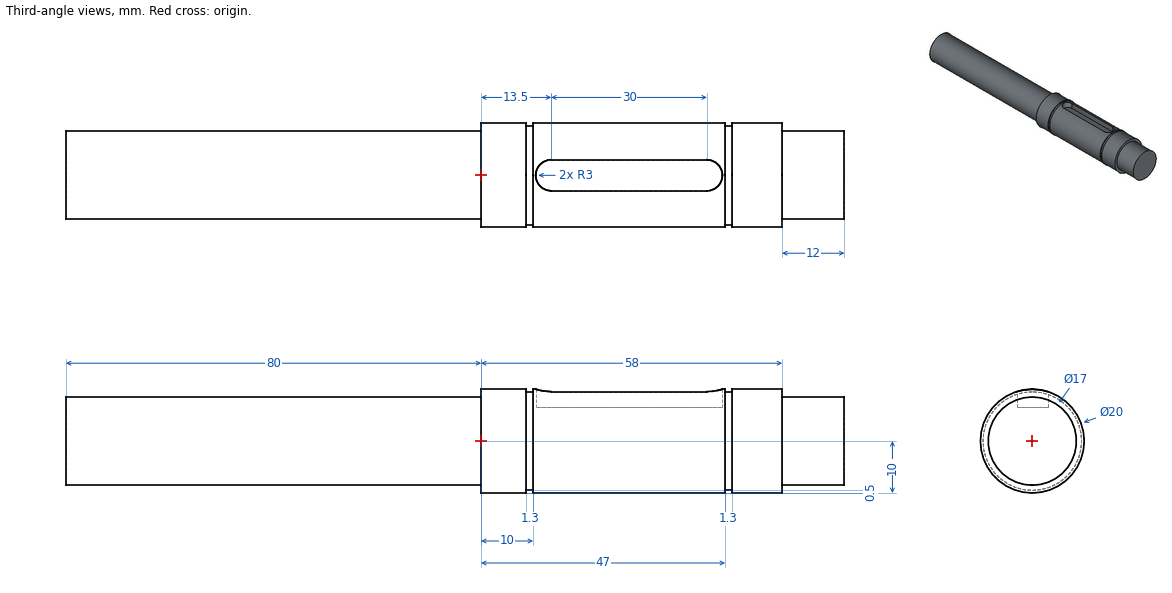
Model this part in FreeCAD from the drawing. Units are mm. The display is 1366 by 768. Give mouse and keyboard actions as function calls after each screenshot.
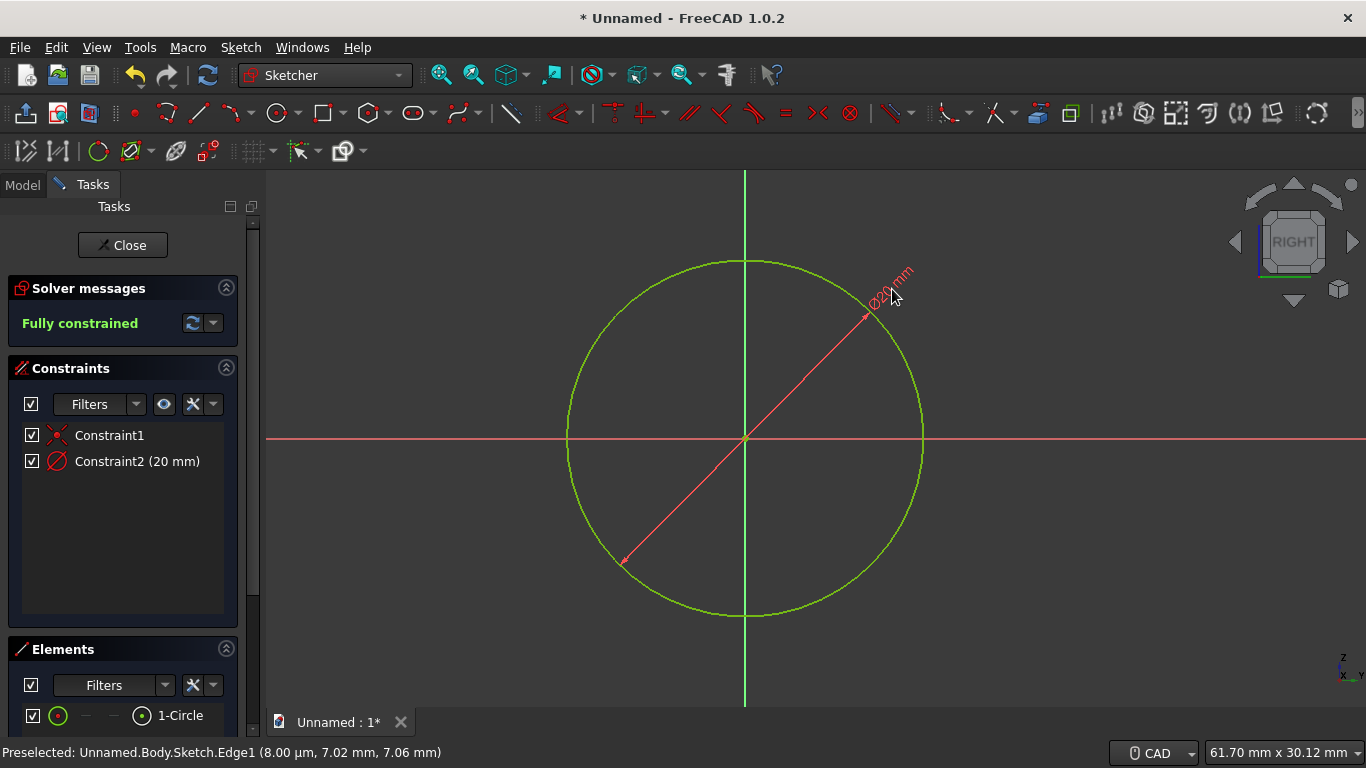
click(123, 245)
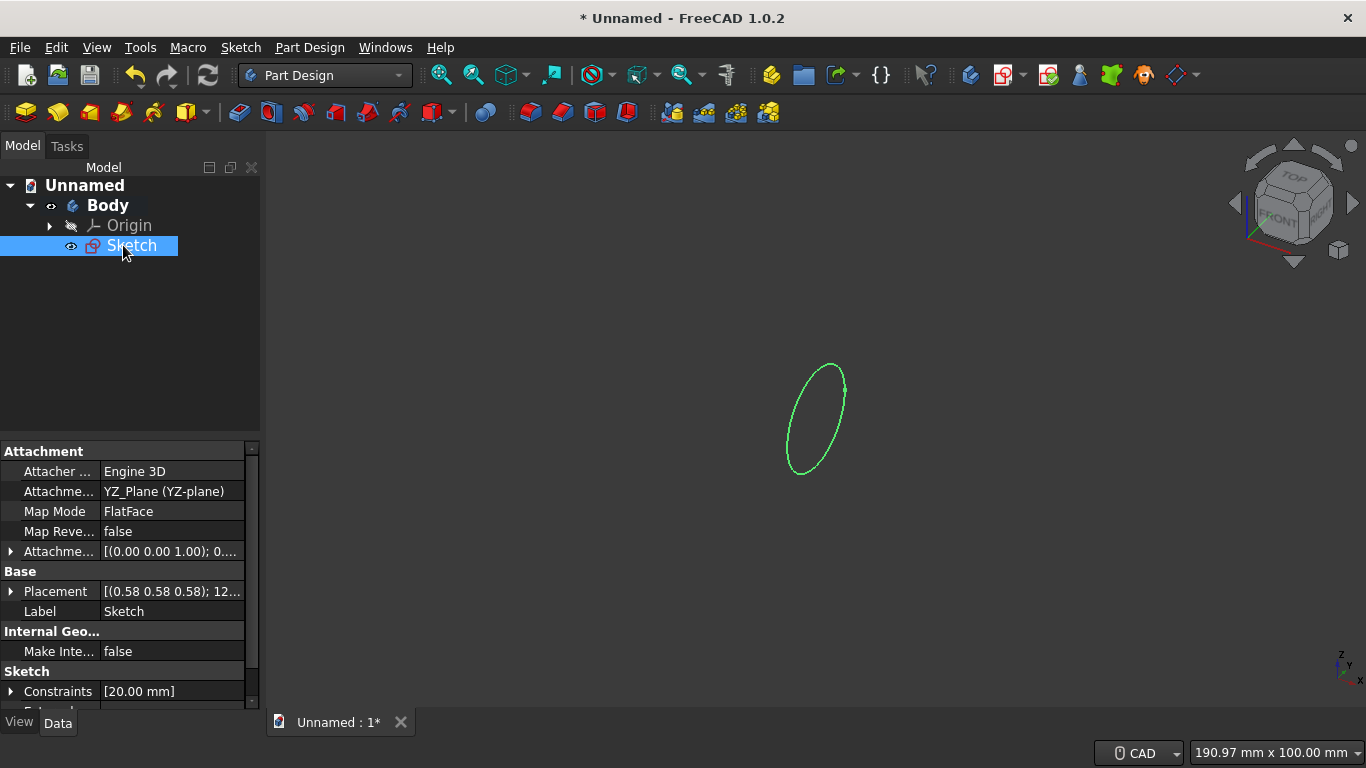
click(26, 112)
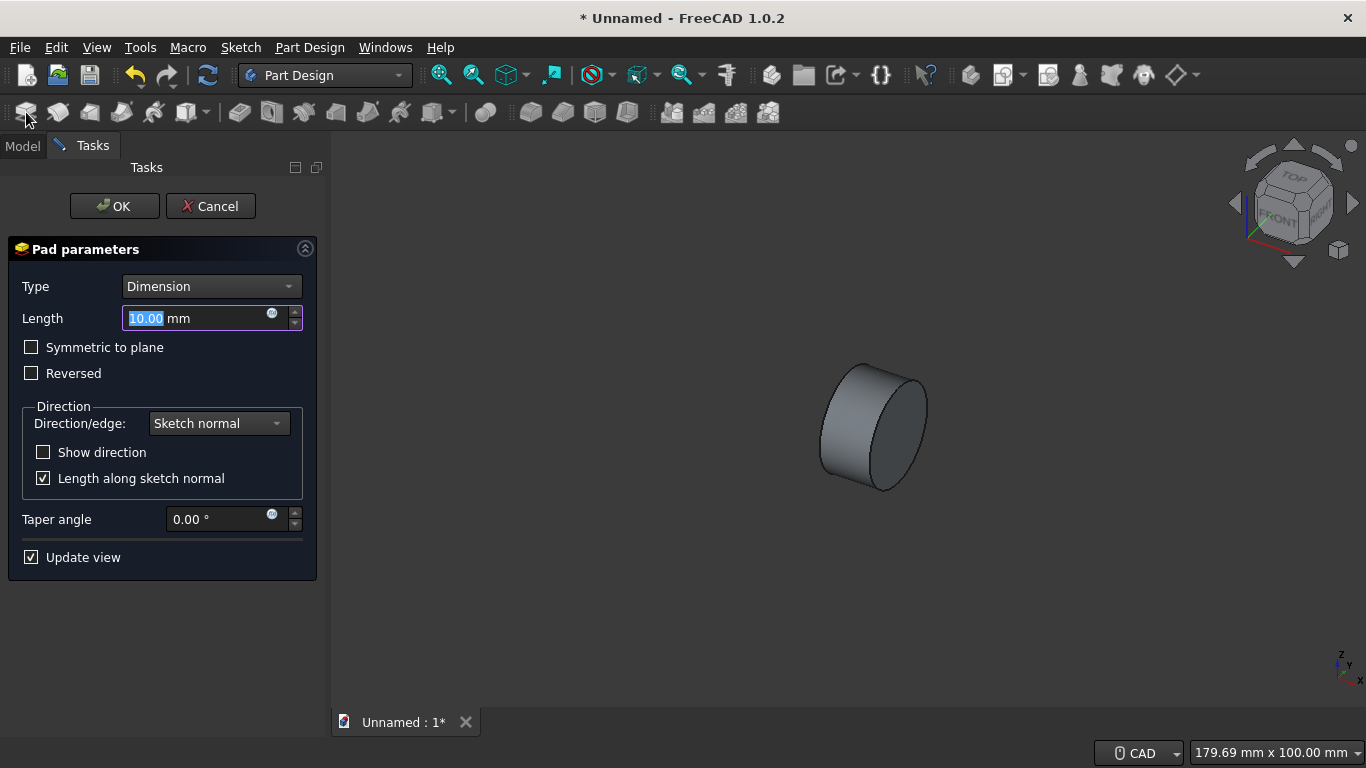
text(58)
key(Tab)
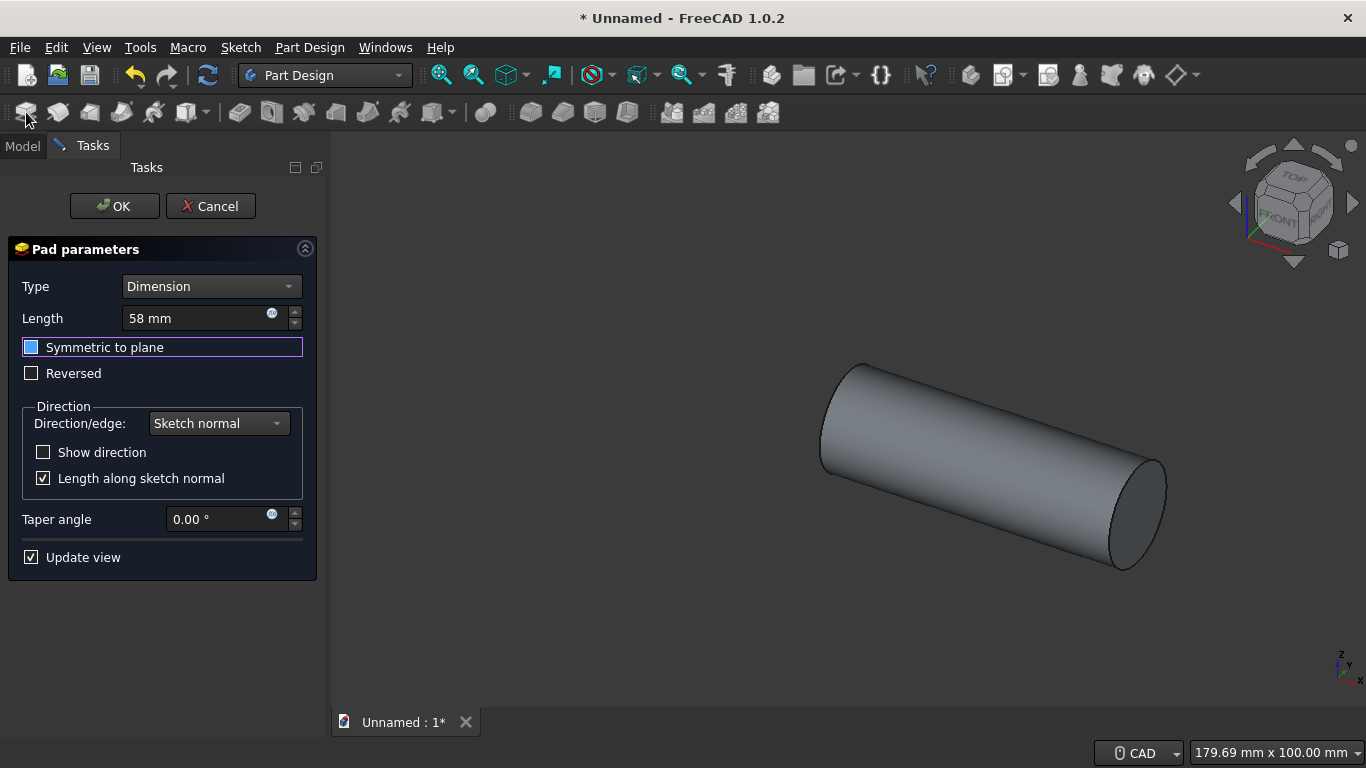
click(115, 206)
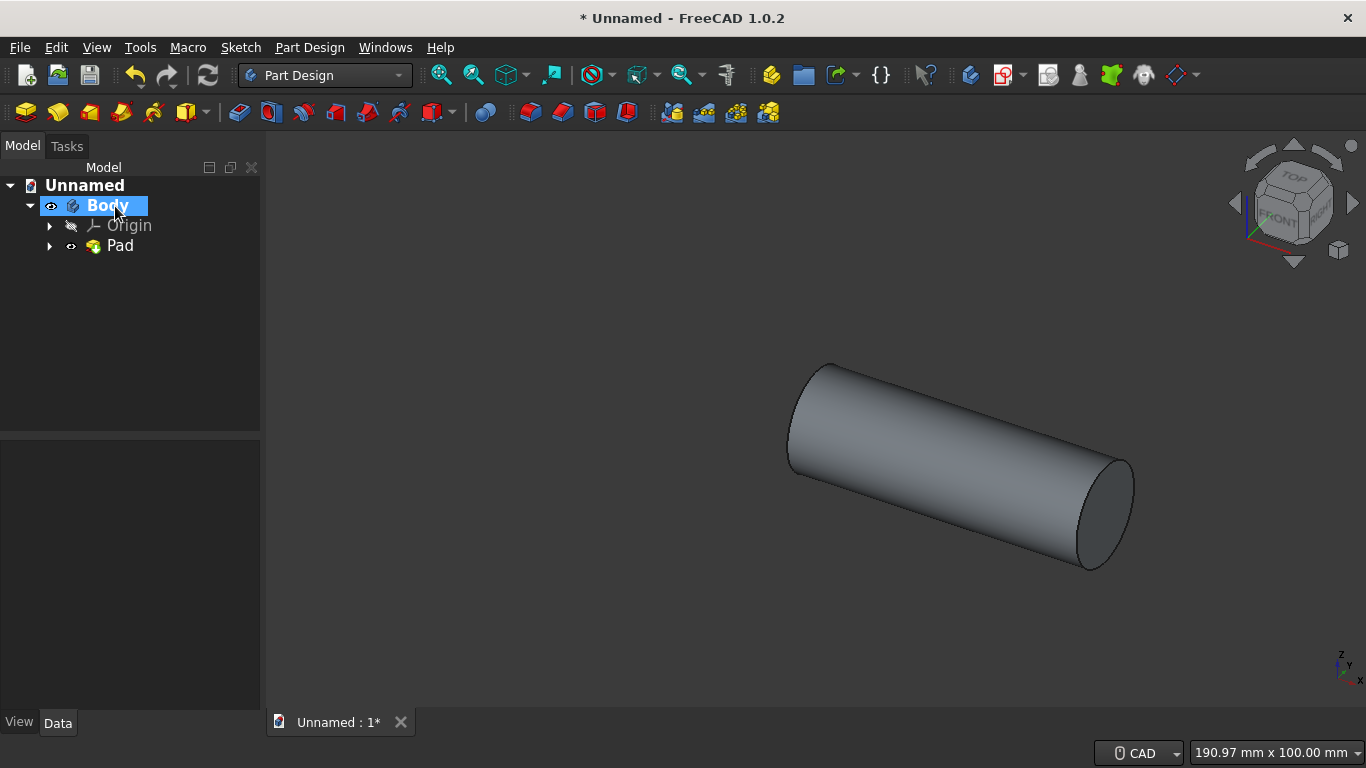
key(v)
key(f)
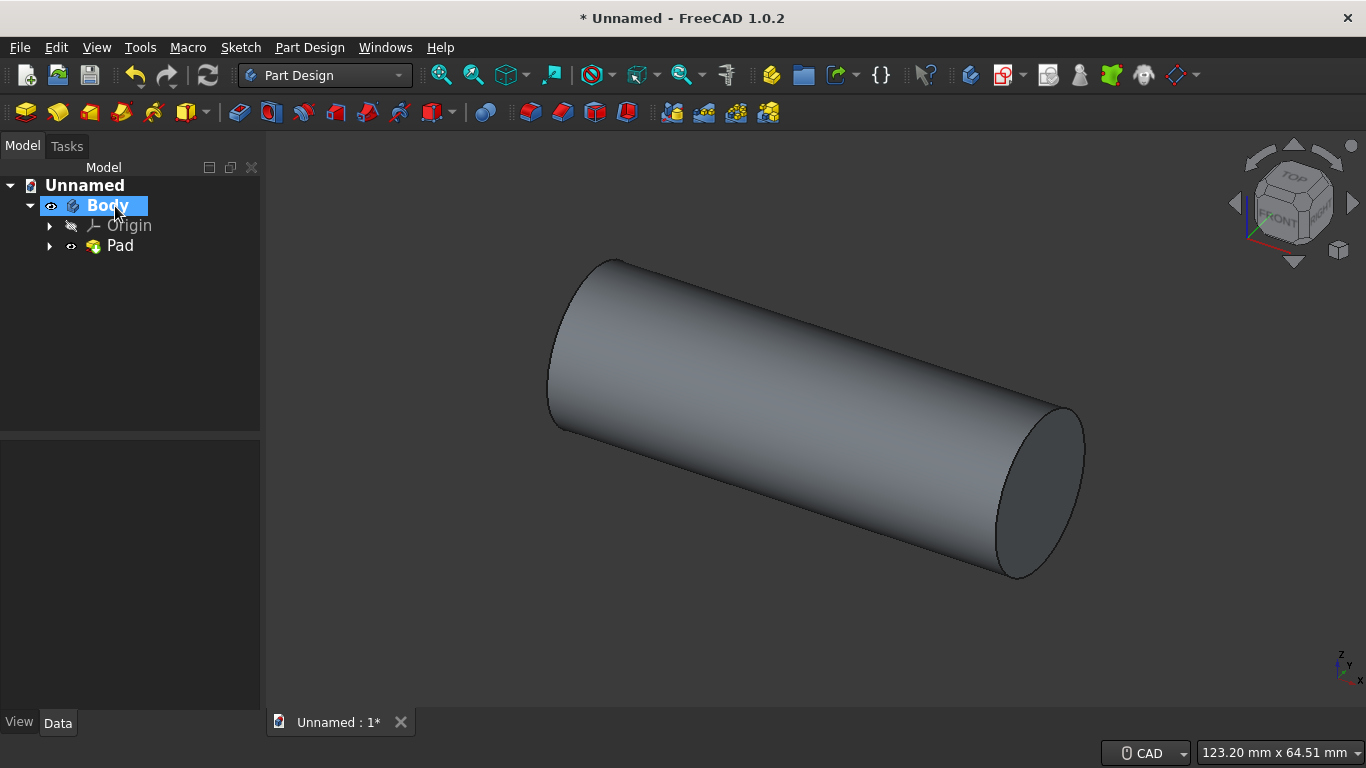
click(1040, 492)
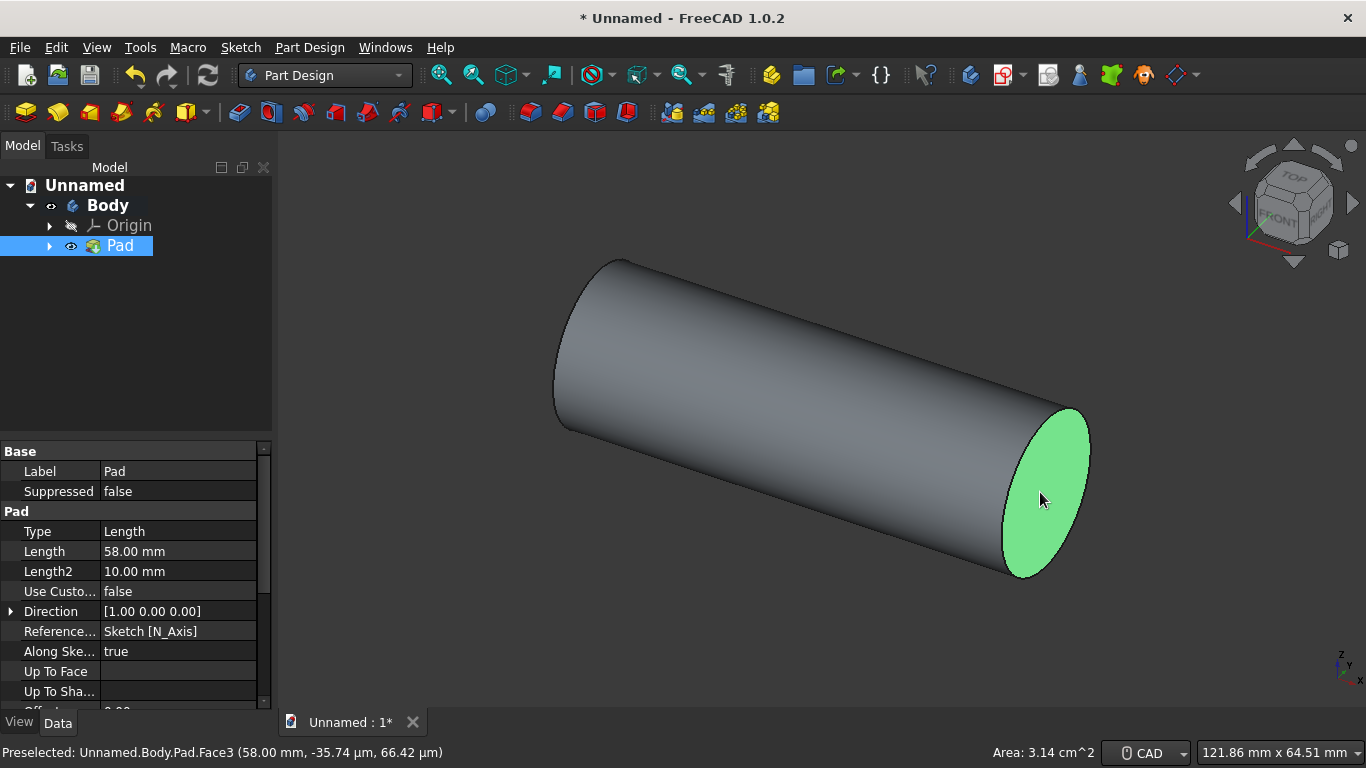
click(1004, 76)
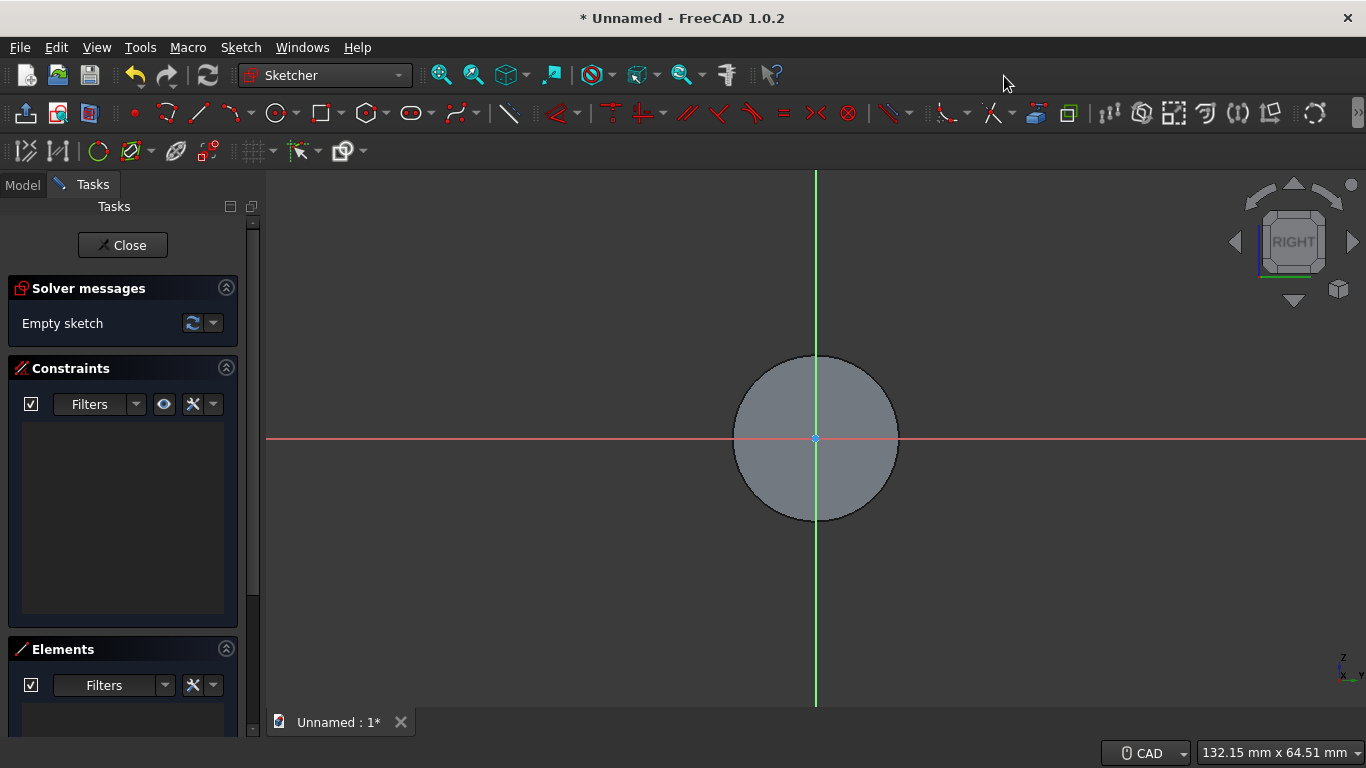
scroll(872, 438, up, 4)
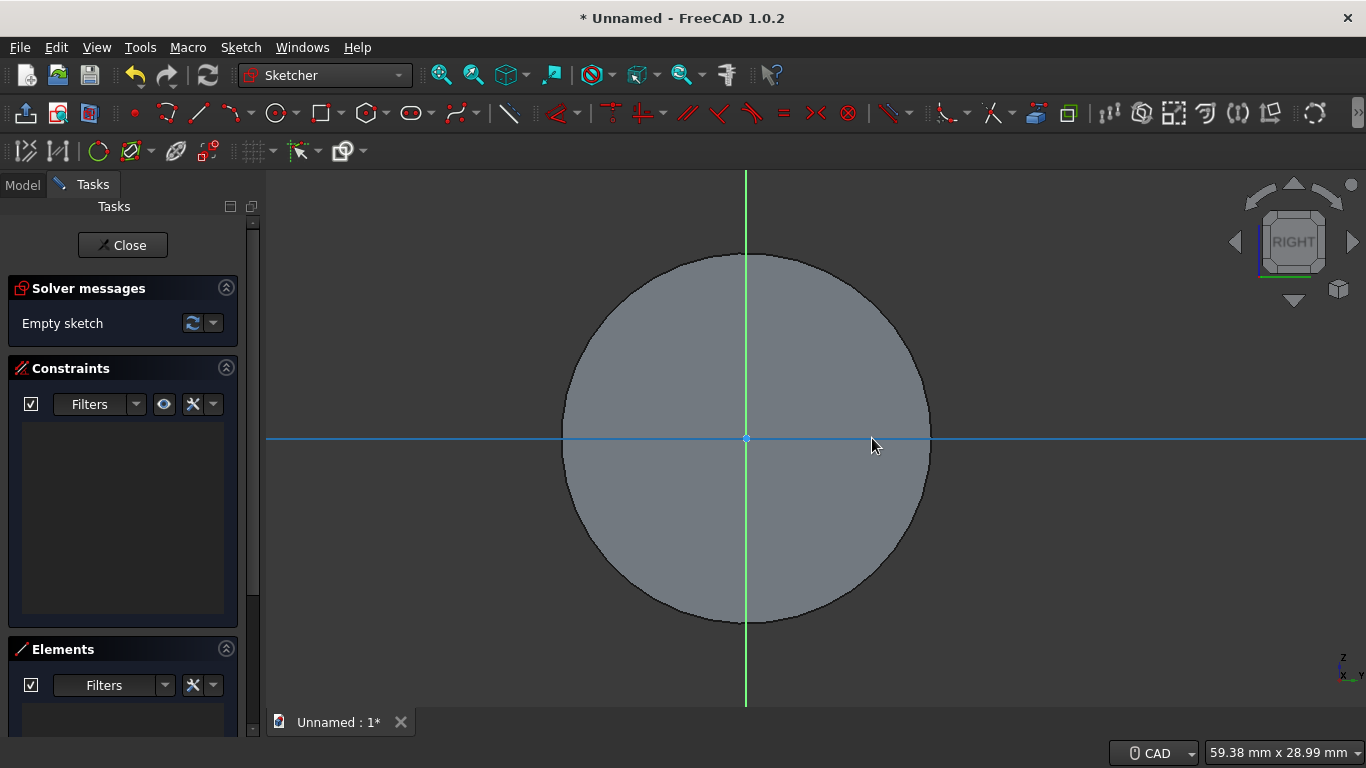
click(276, 114)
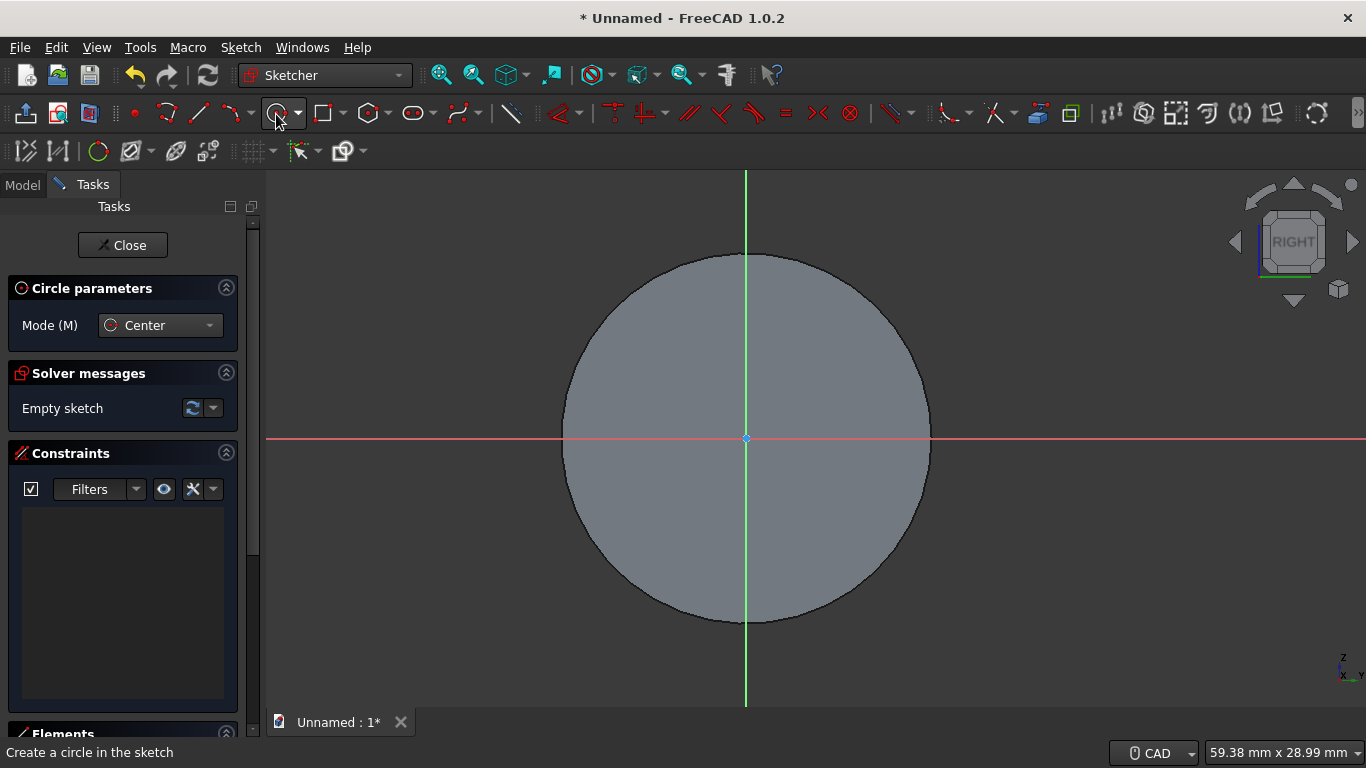
click(746, 438)
click(858, 327)
key(Escape)